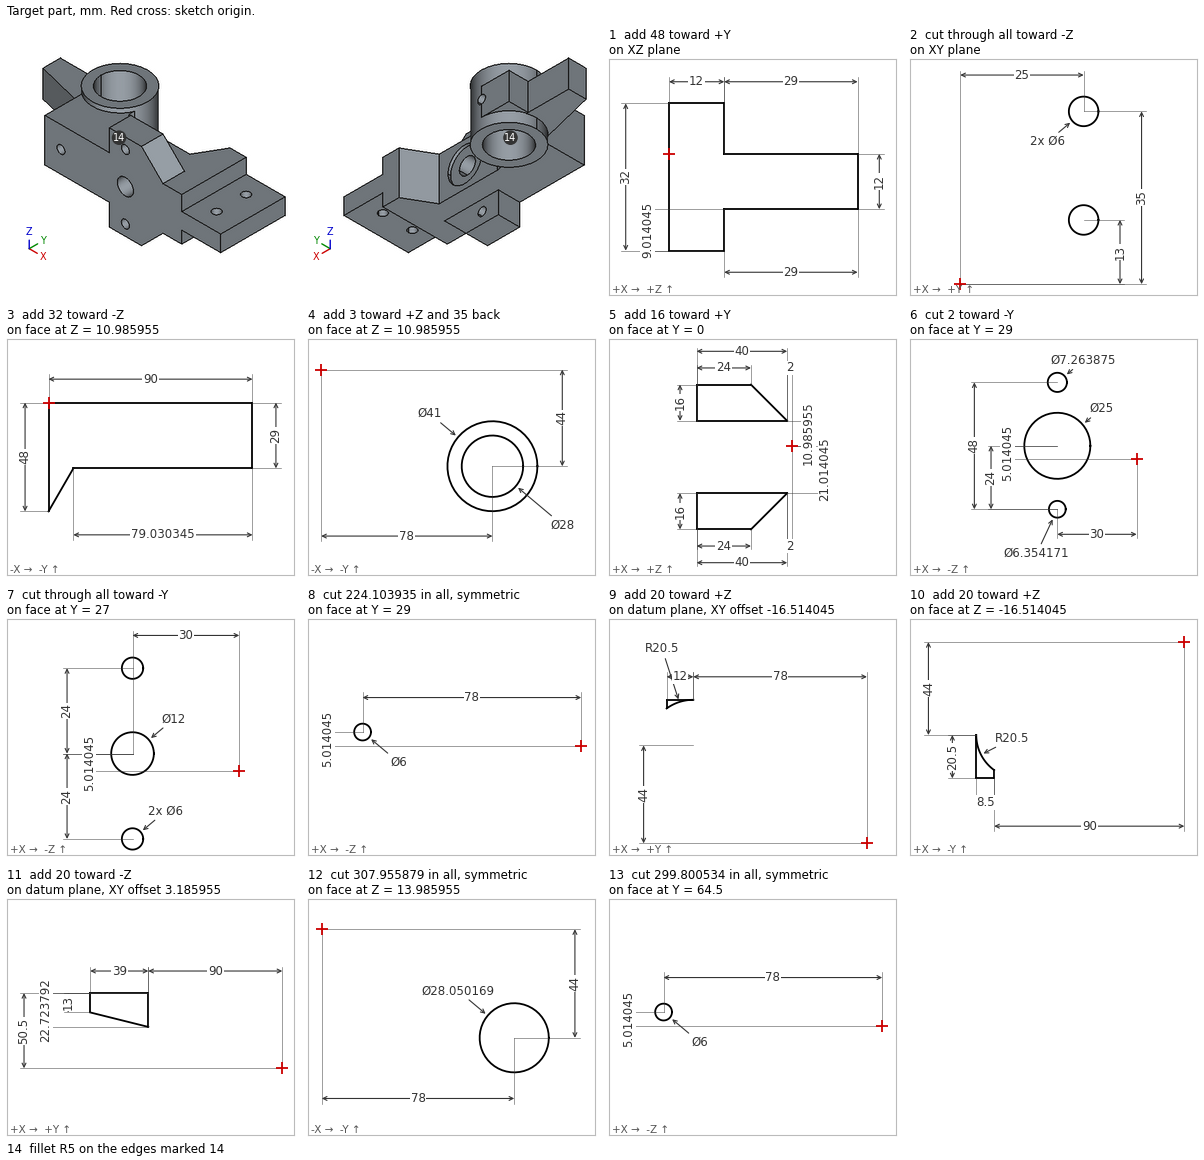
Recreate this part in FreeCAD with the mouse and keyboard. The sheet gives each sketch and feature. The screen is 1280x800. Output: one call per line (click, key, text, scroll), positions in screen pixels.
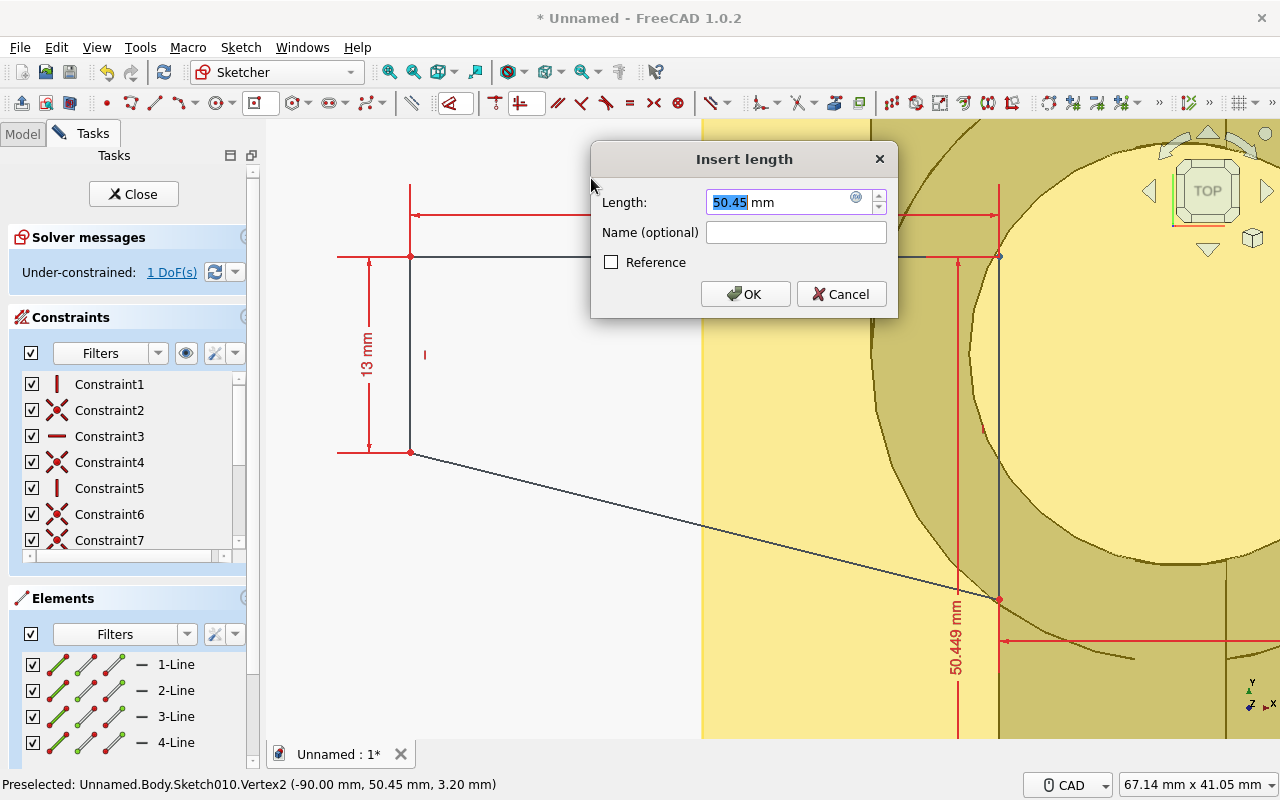
text(50.5)
key(Return)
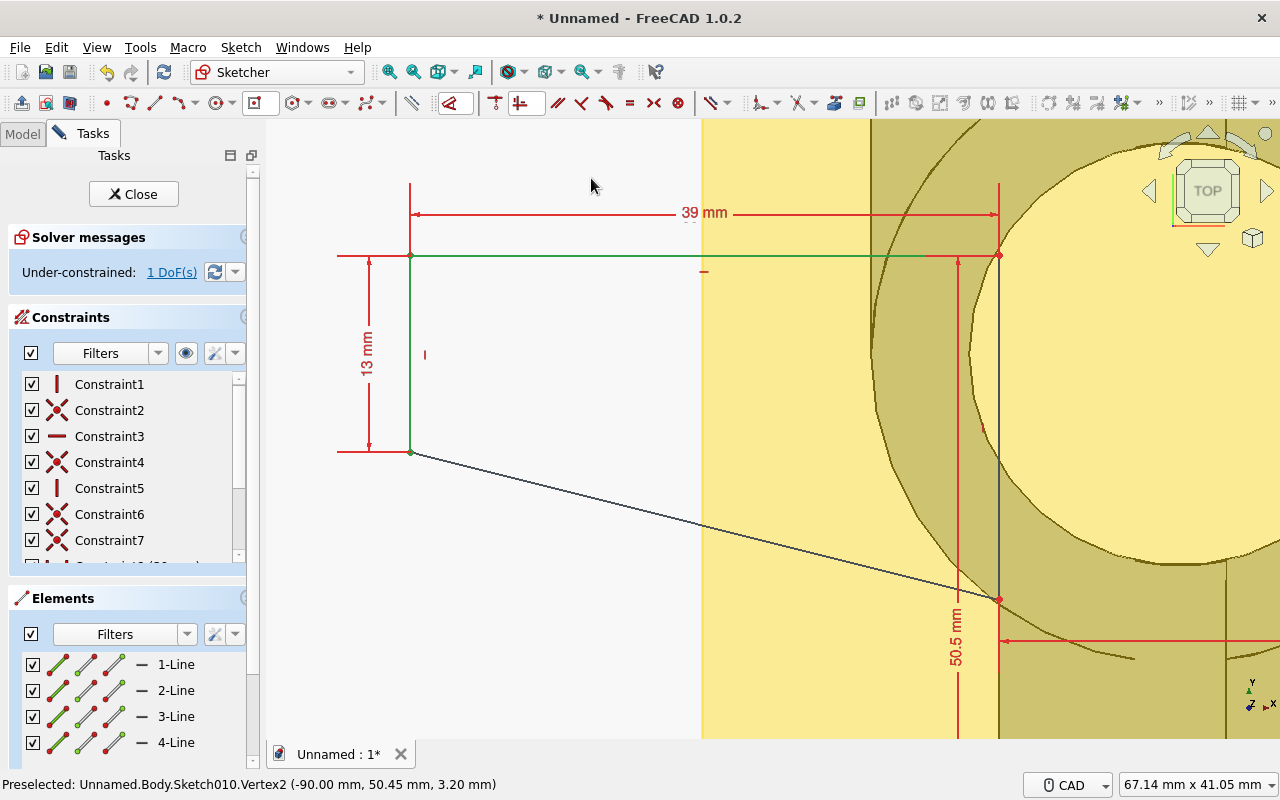
click(999, 497)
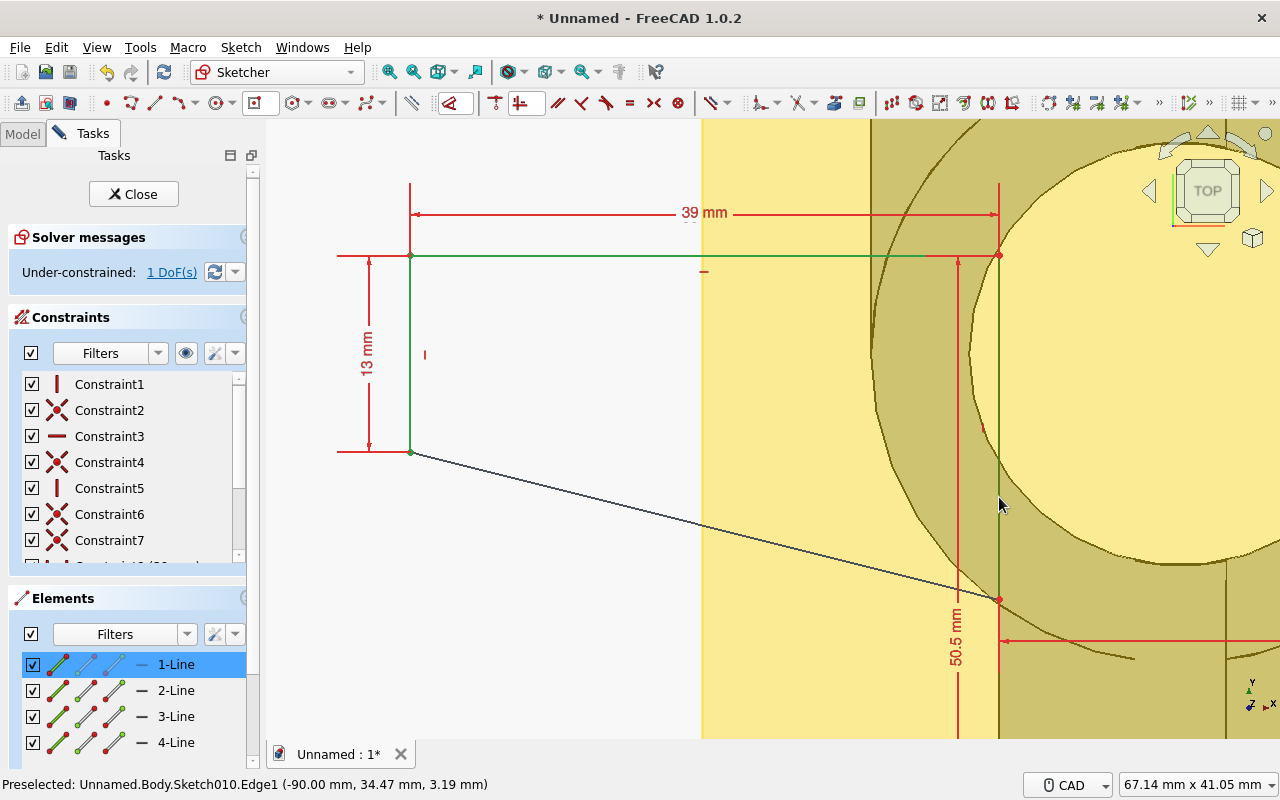
key(i)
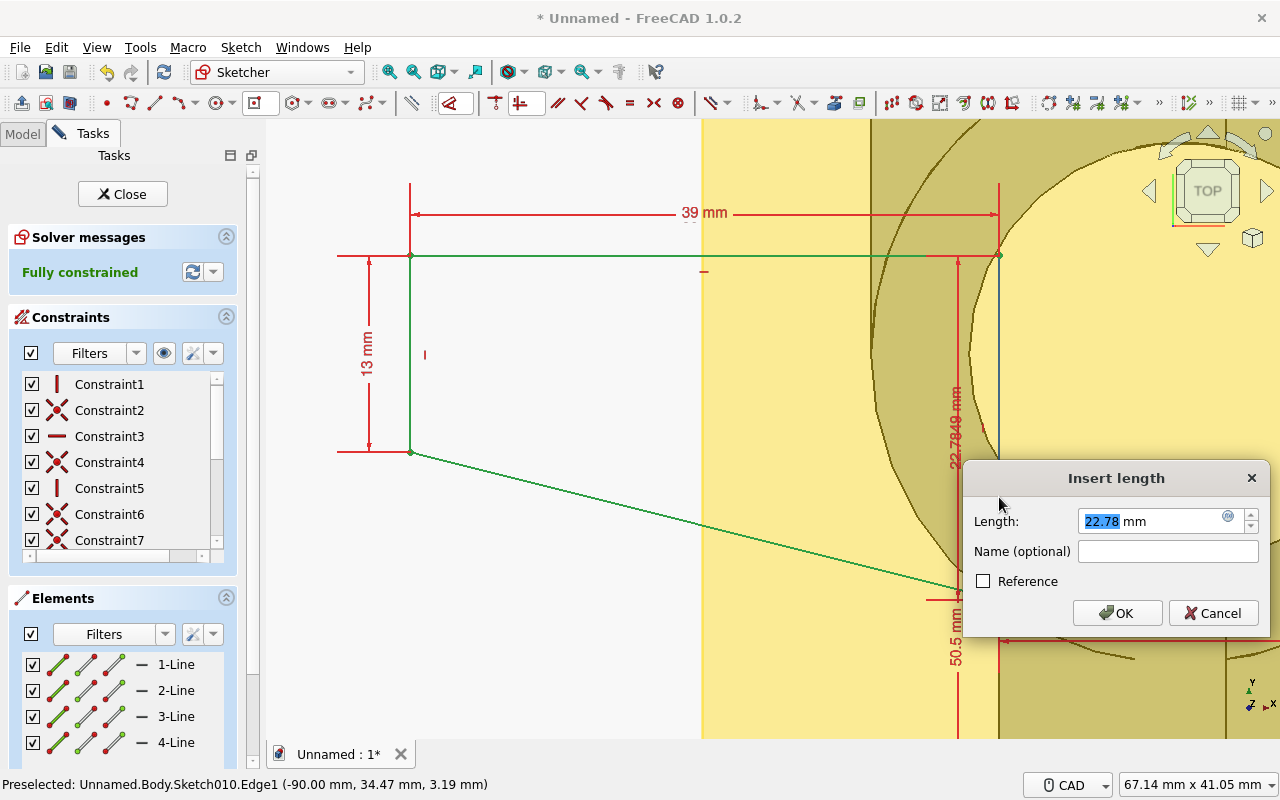
text(22.723792)
key(Return)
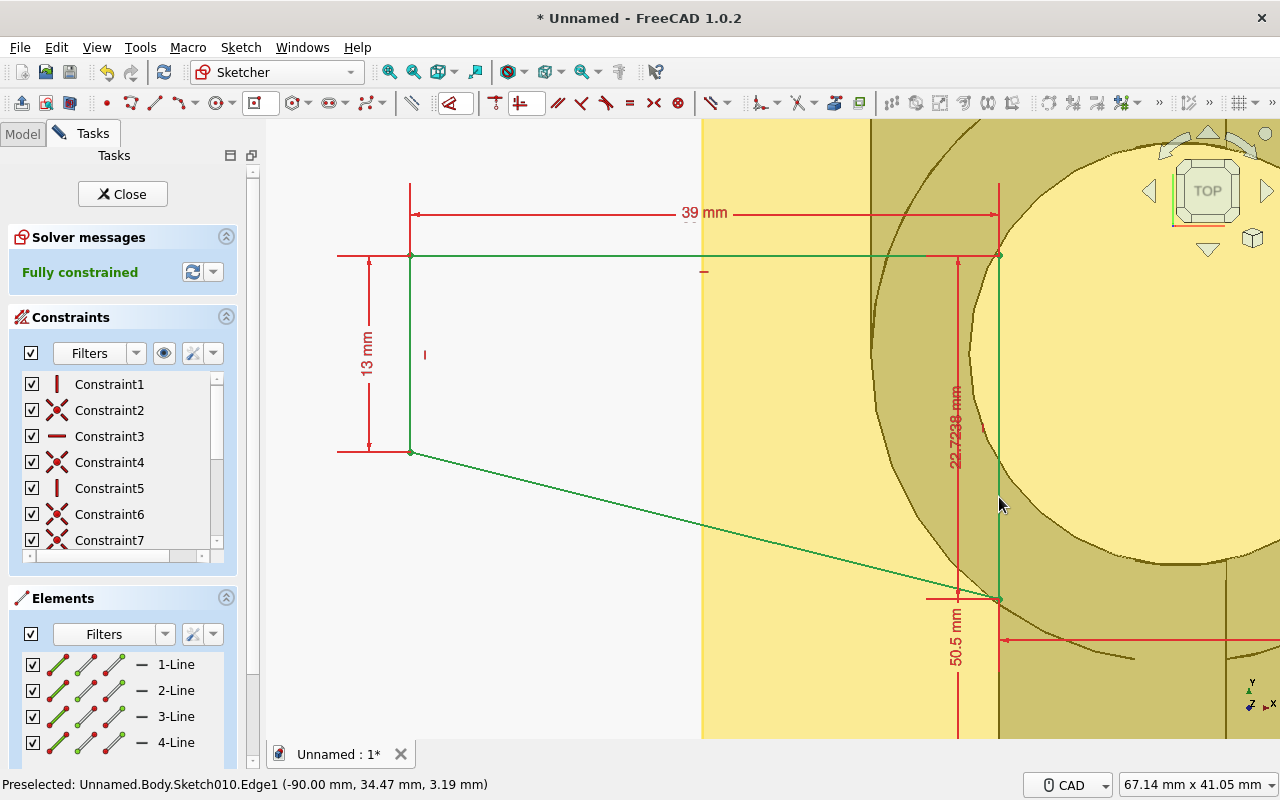
click(123, 194)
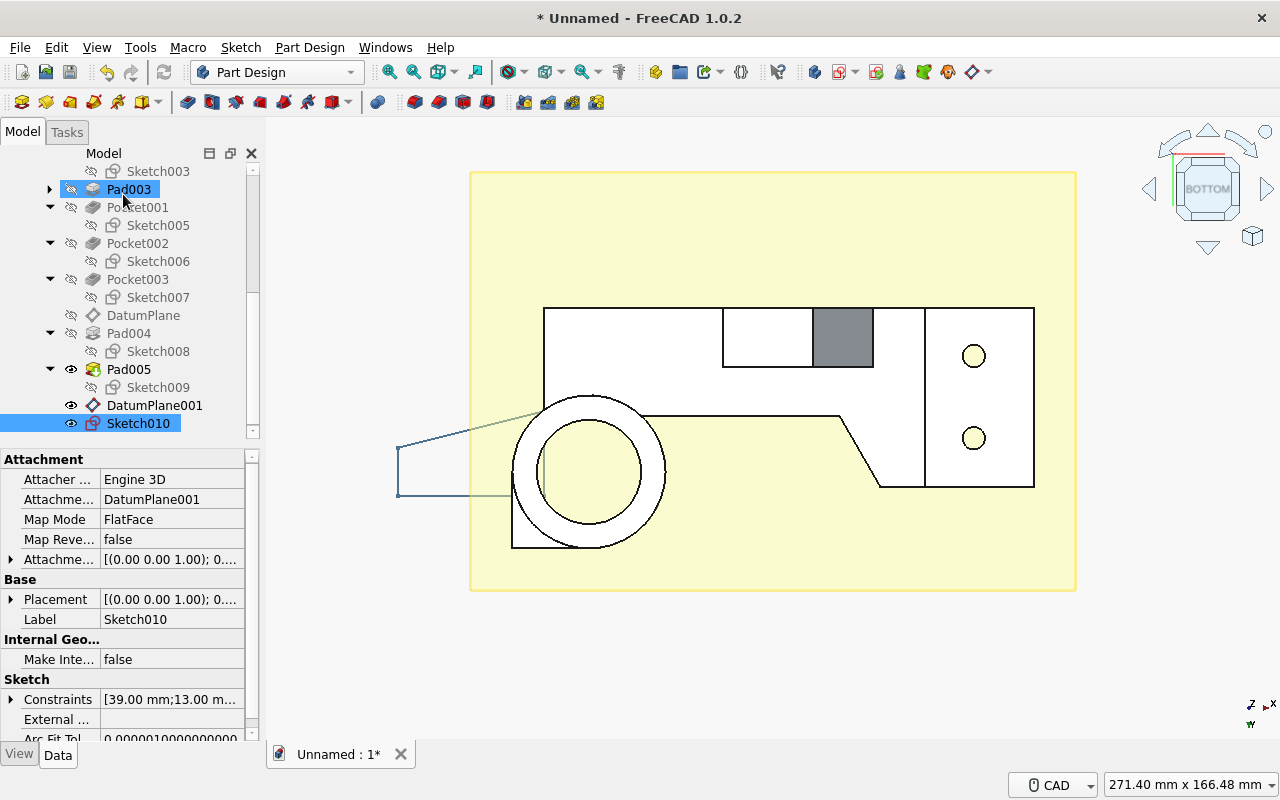
click(22, 102)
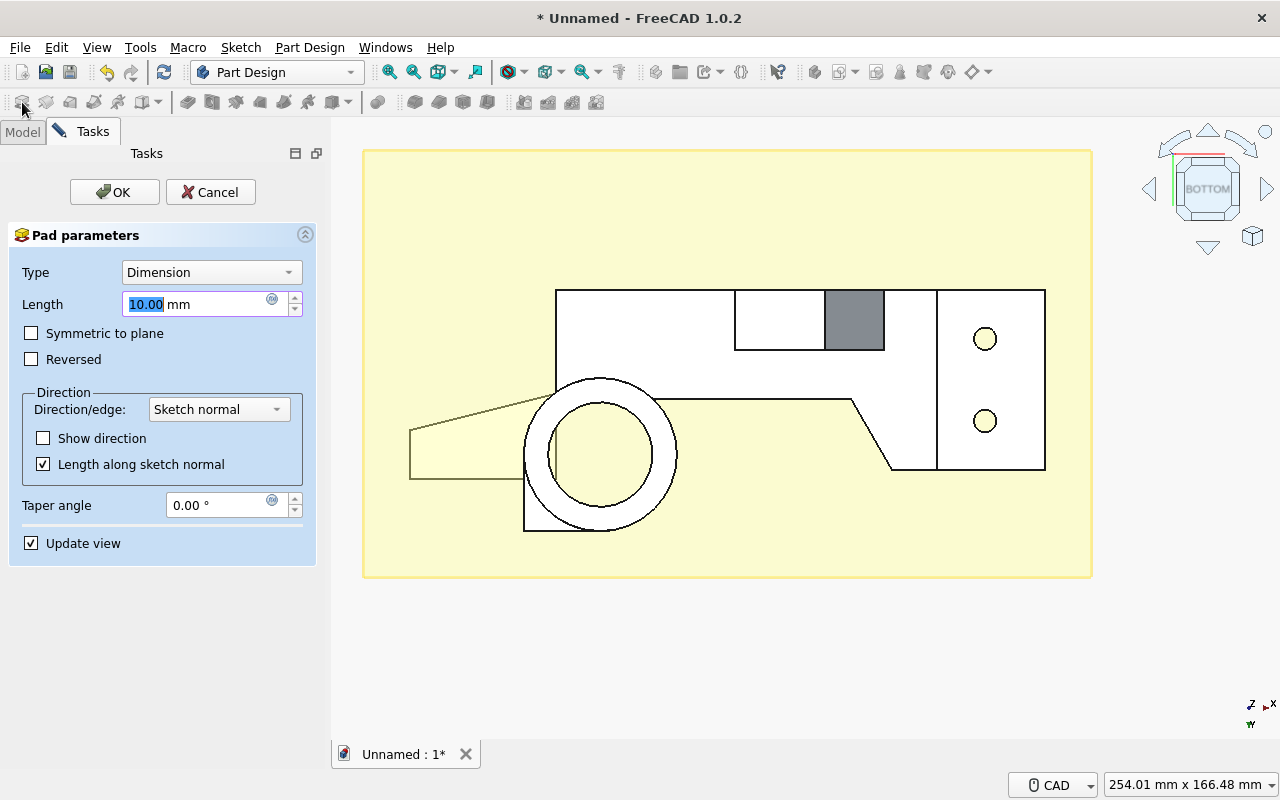
text(20)
key(Tab)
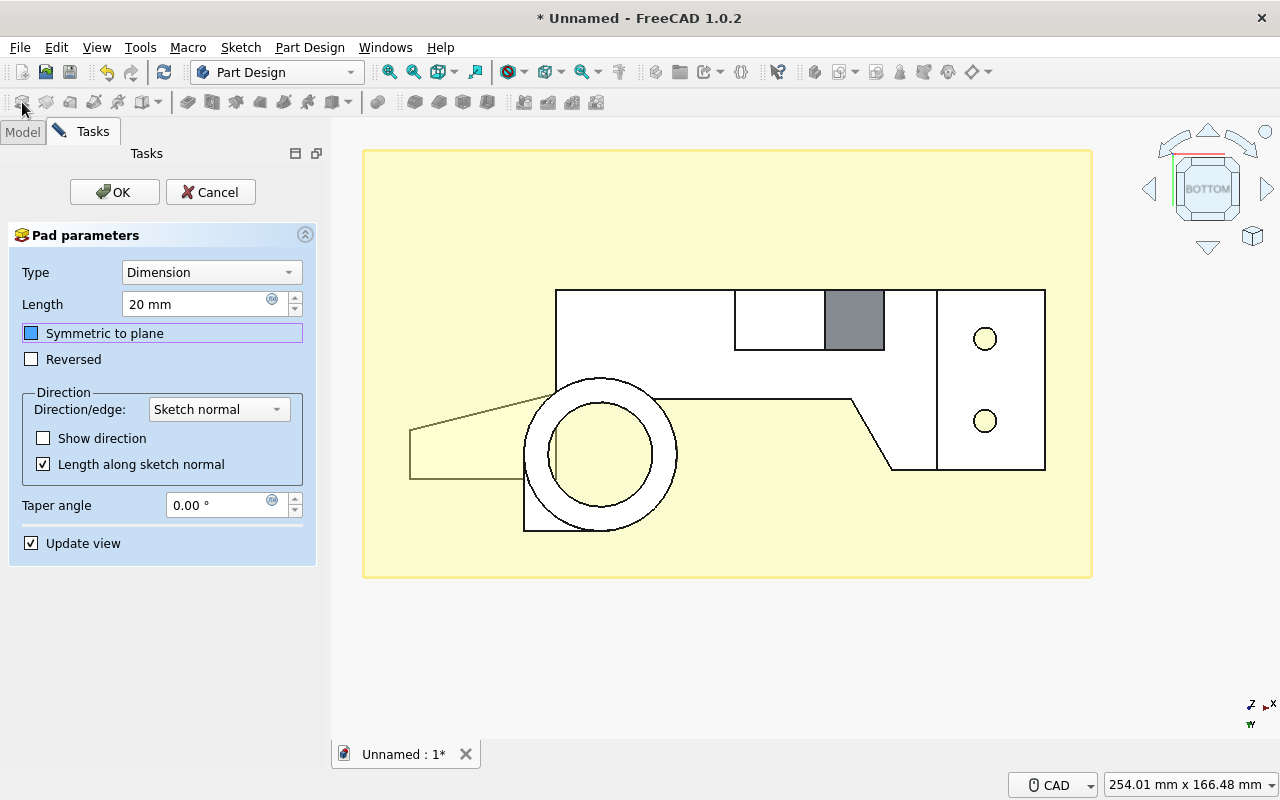
click(30, 359)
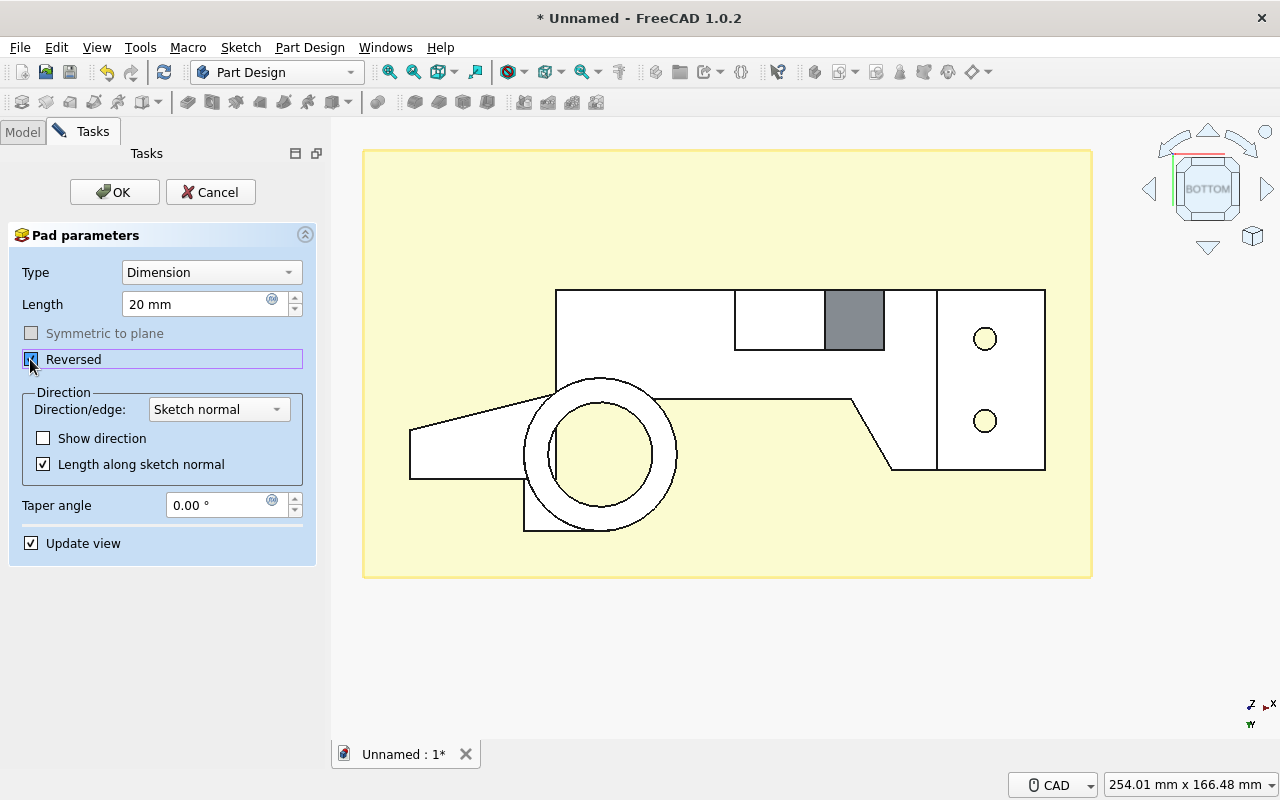
click(115, 192)